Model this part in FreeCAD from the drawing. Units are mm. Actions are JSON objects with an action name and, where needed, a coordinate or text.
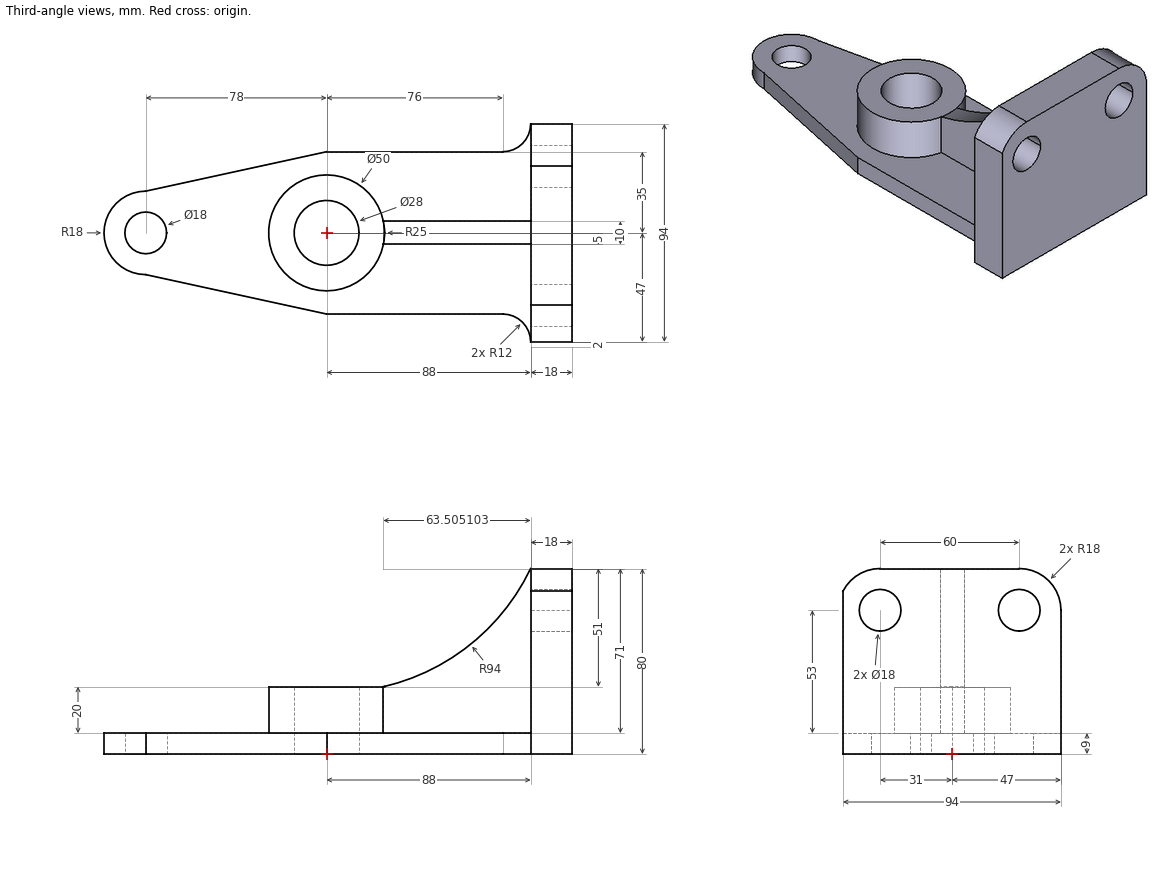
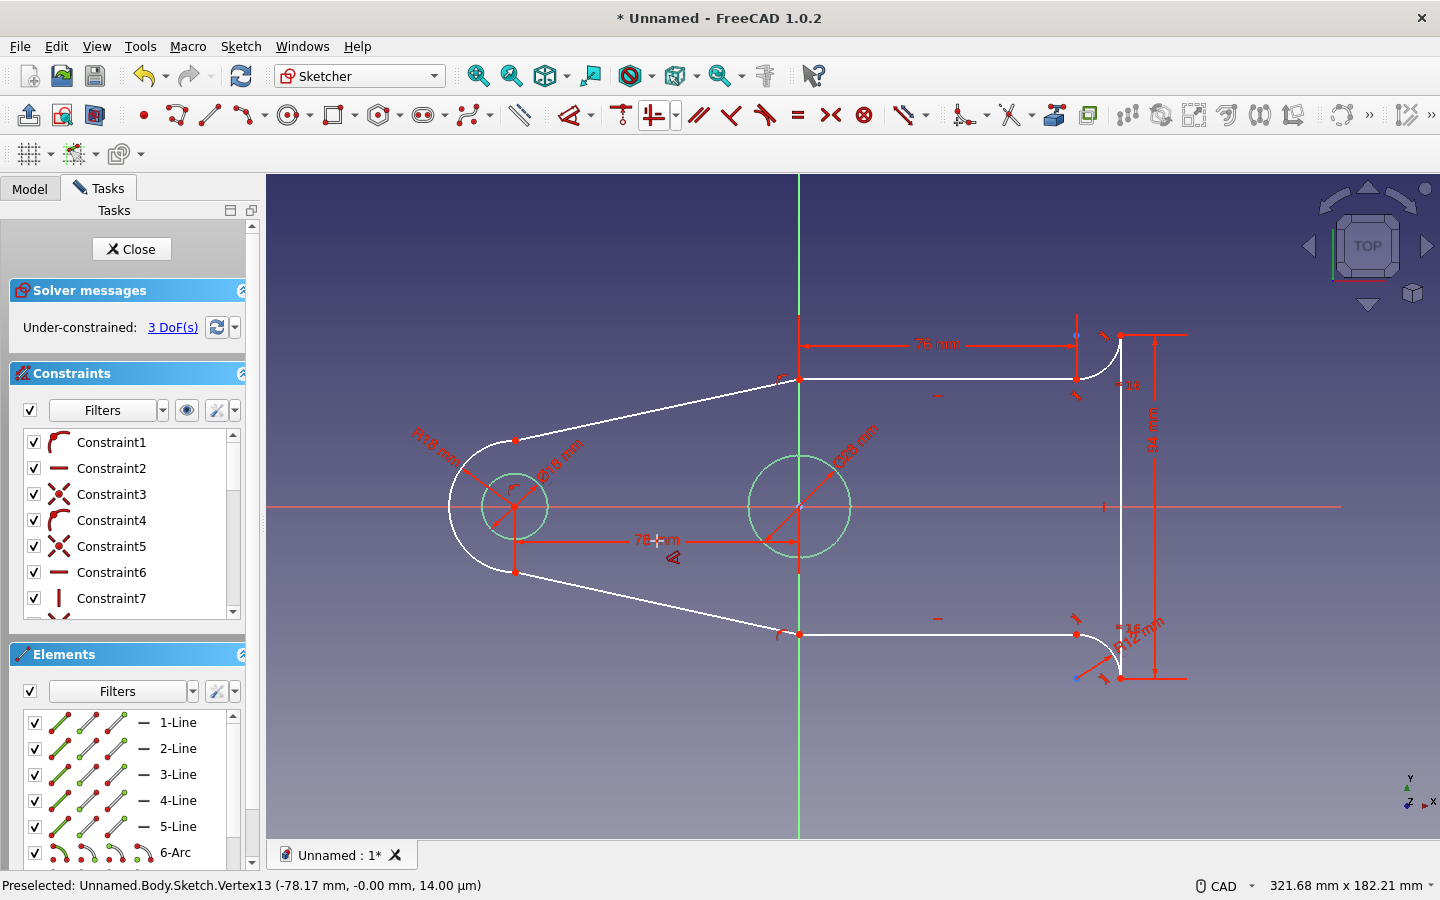
{"action": "left_click", "coordinate": [1077, 379]}
{"action": "left_click", "coordinate": [765, 443]}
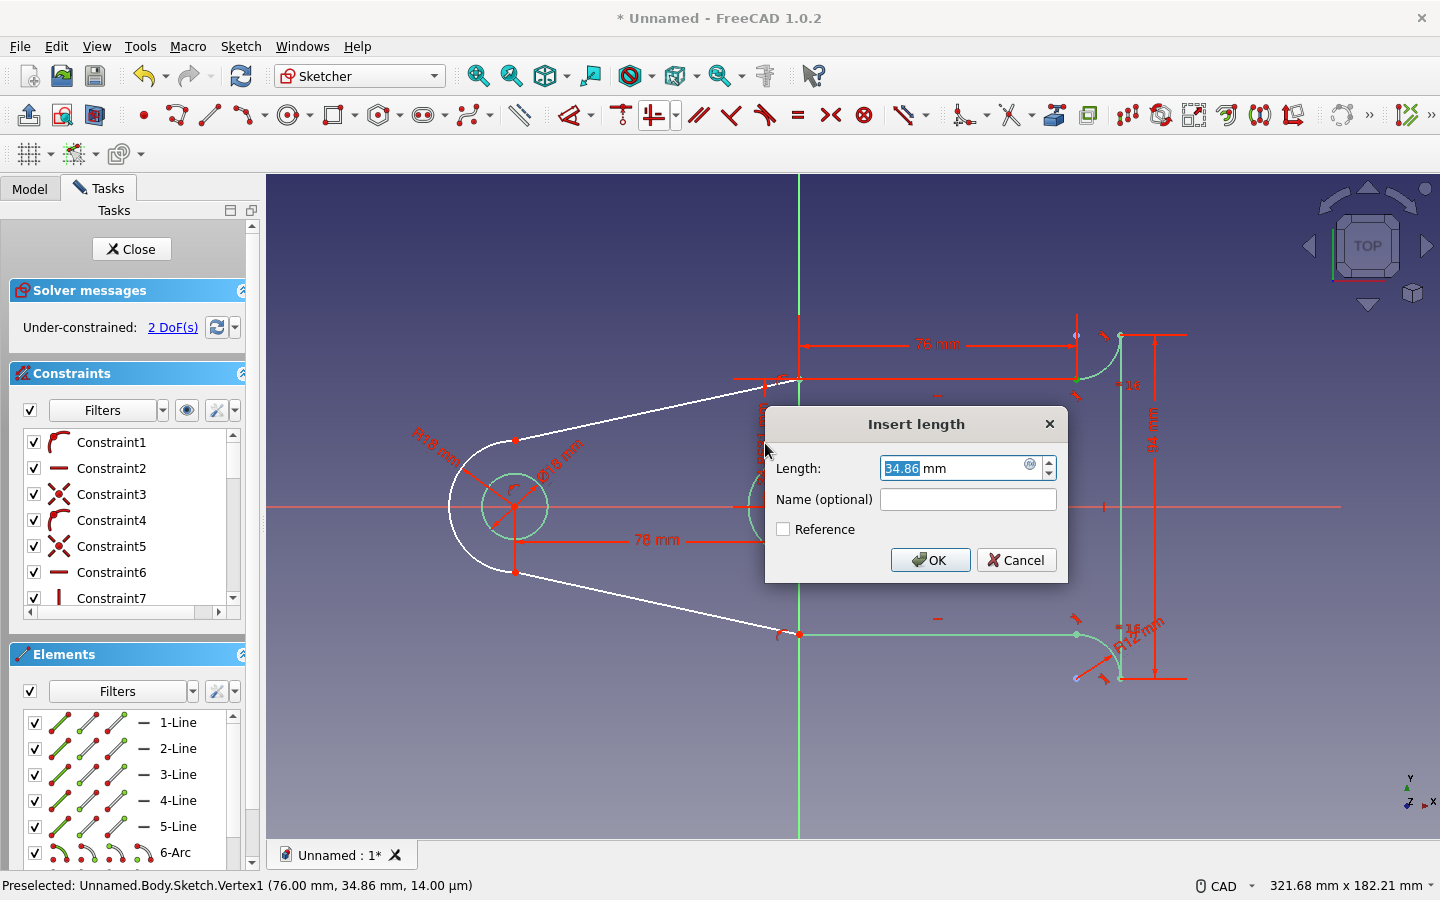
{"action": "type", "text": "35"}
{"action": "key", "text": "Return"}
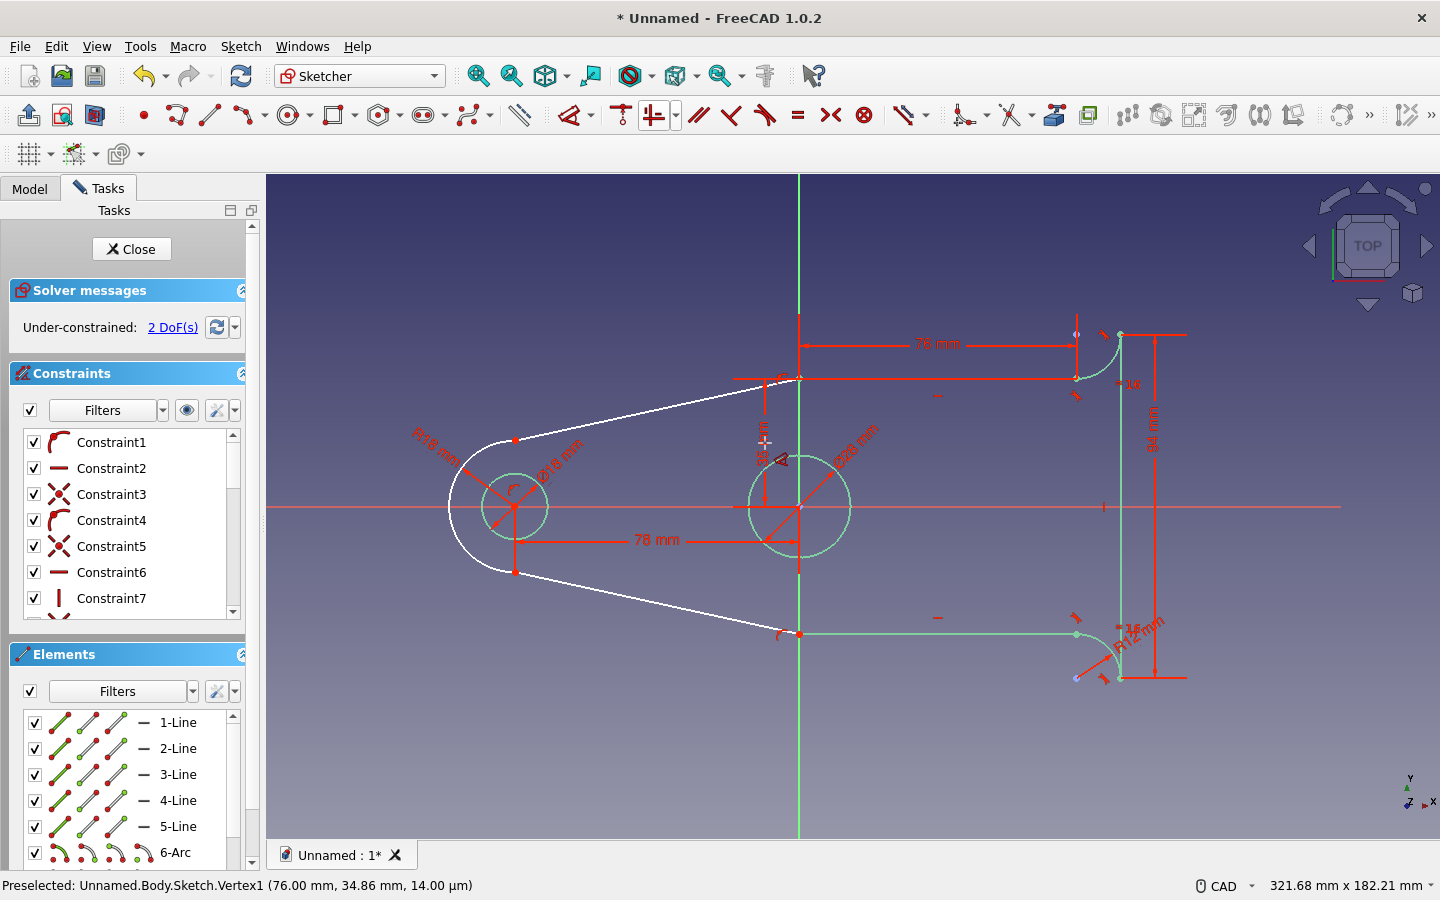
{"action": "left_click", "coordinate": [515, 441]}
{"action": "left_click", "coordinate": [592, 407]}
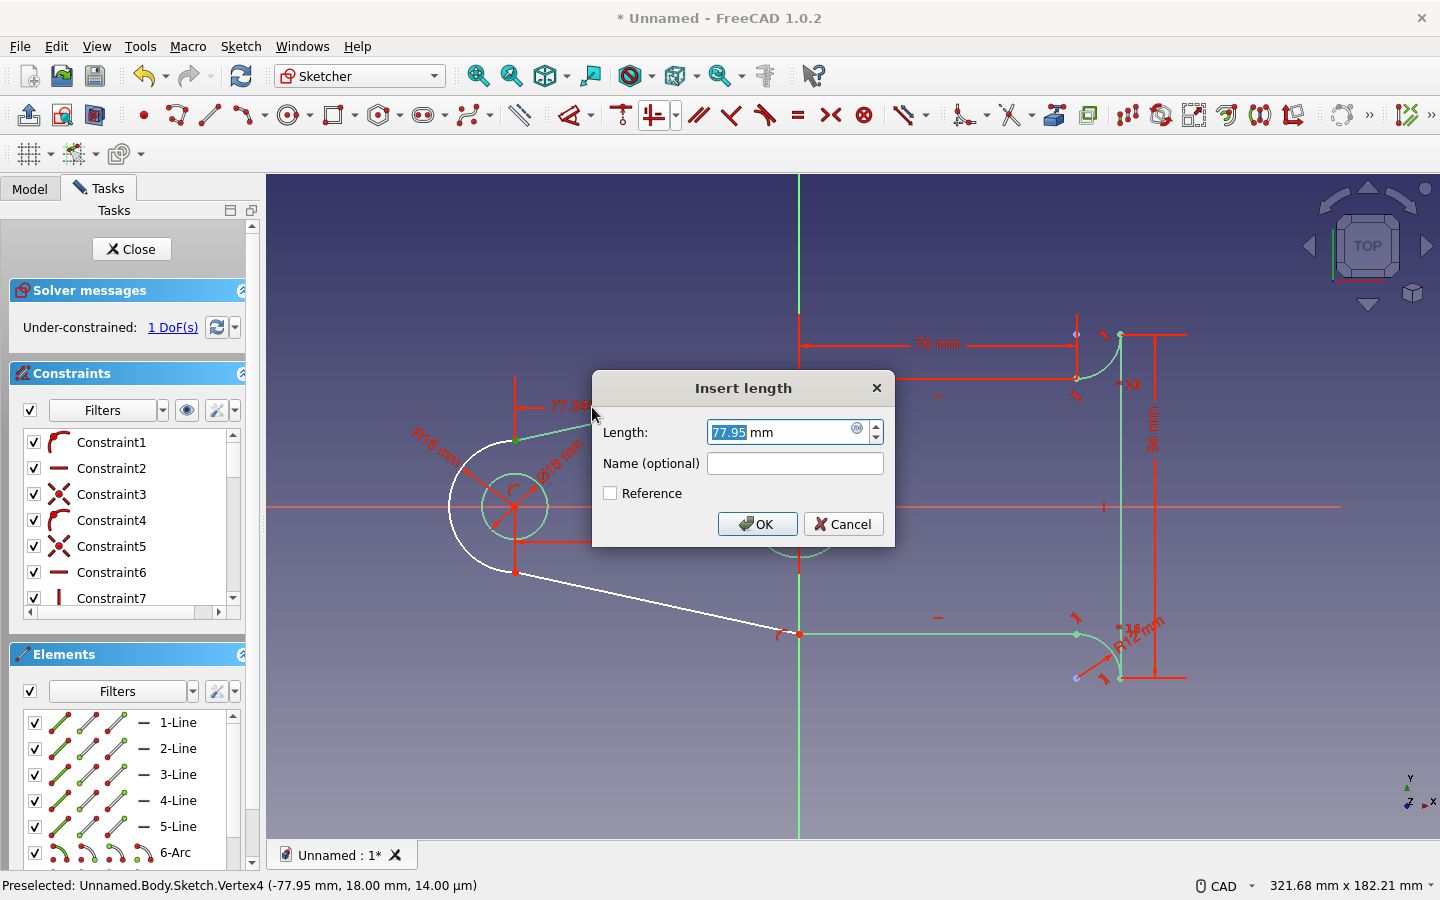
{"action": "type", "text": "78"}
{"action": "key", "text": "Return"}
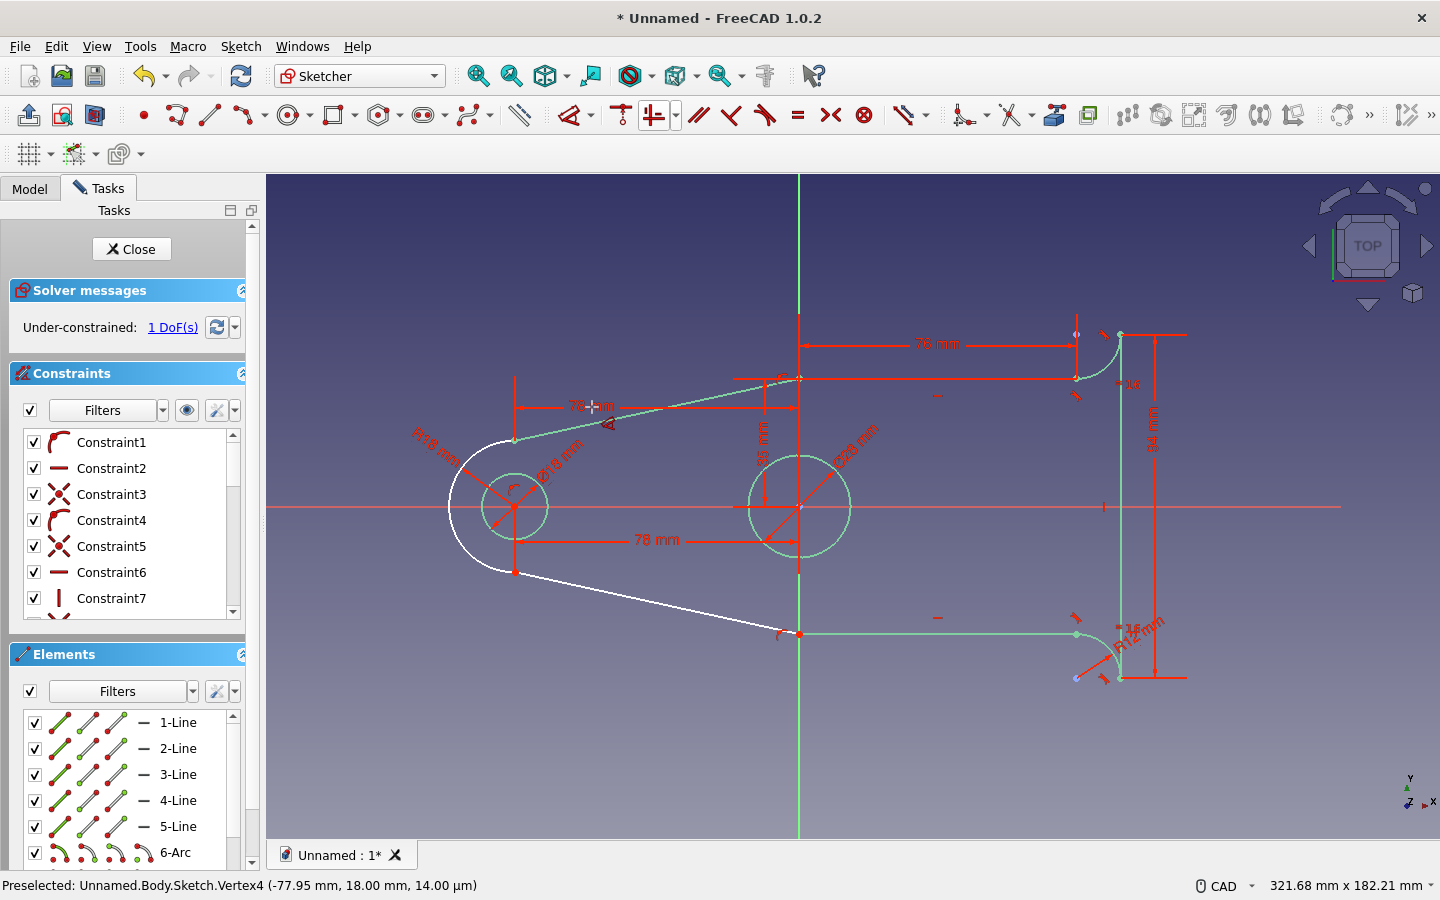
{"action": "left_click", "coordinate": [515, 572]}
{"action": "left_click", "coordinate": [592, 606]}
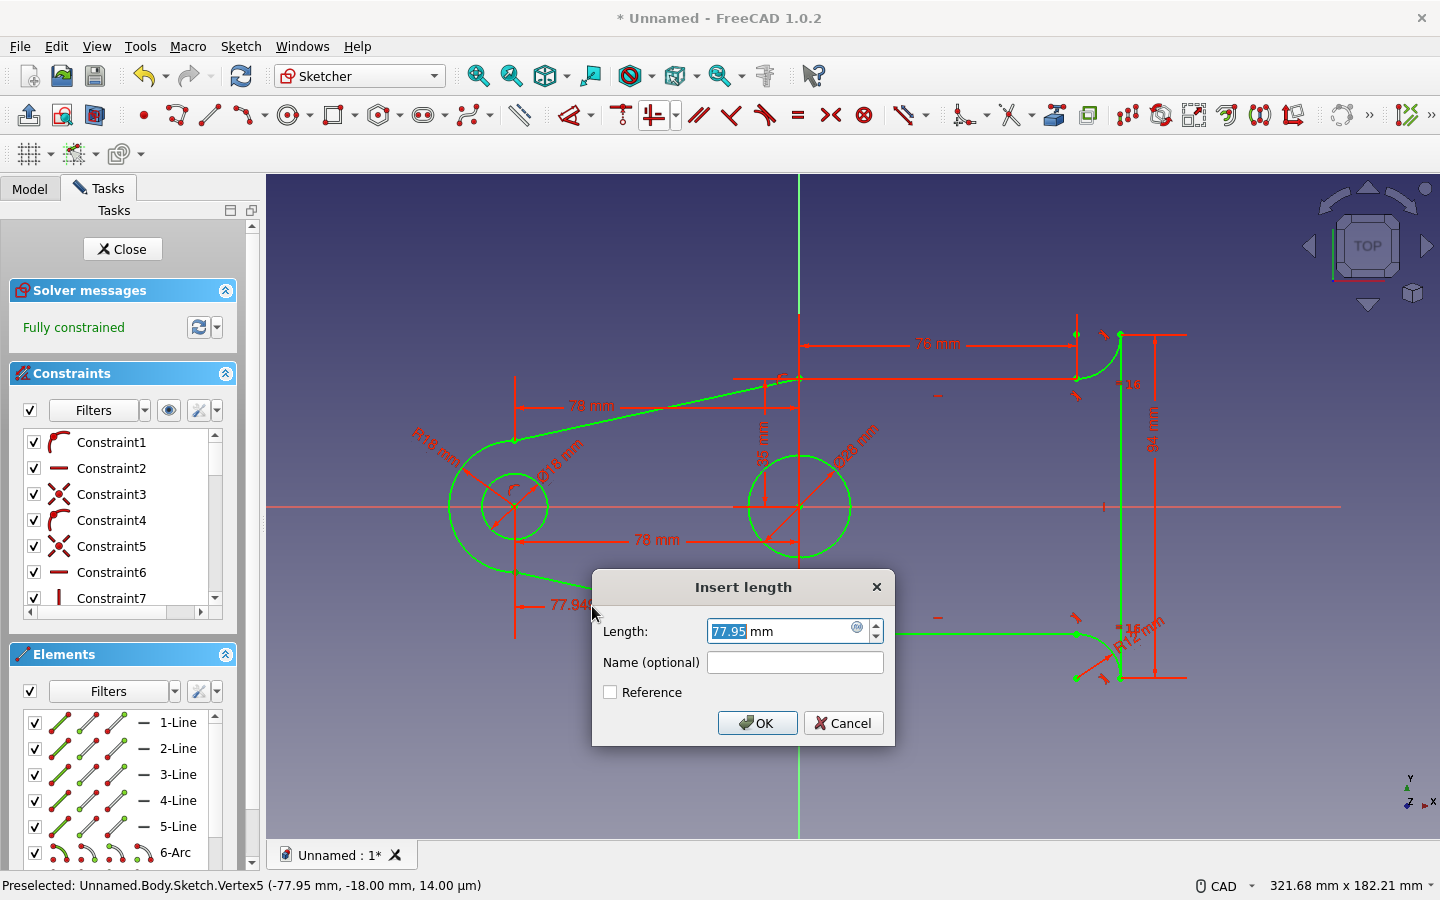
{"action": "type", "text": "78"}
{"action": "key", "text": "Return"}
{"action": "key", "text": "Escape"}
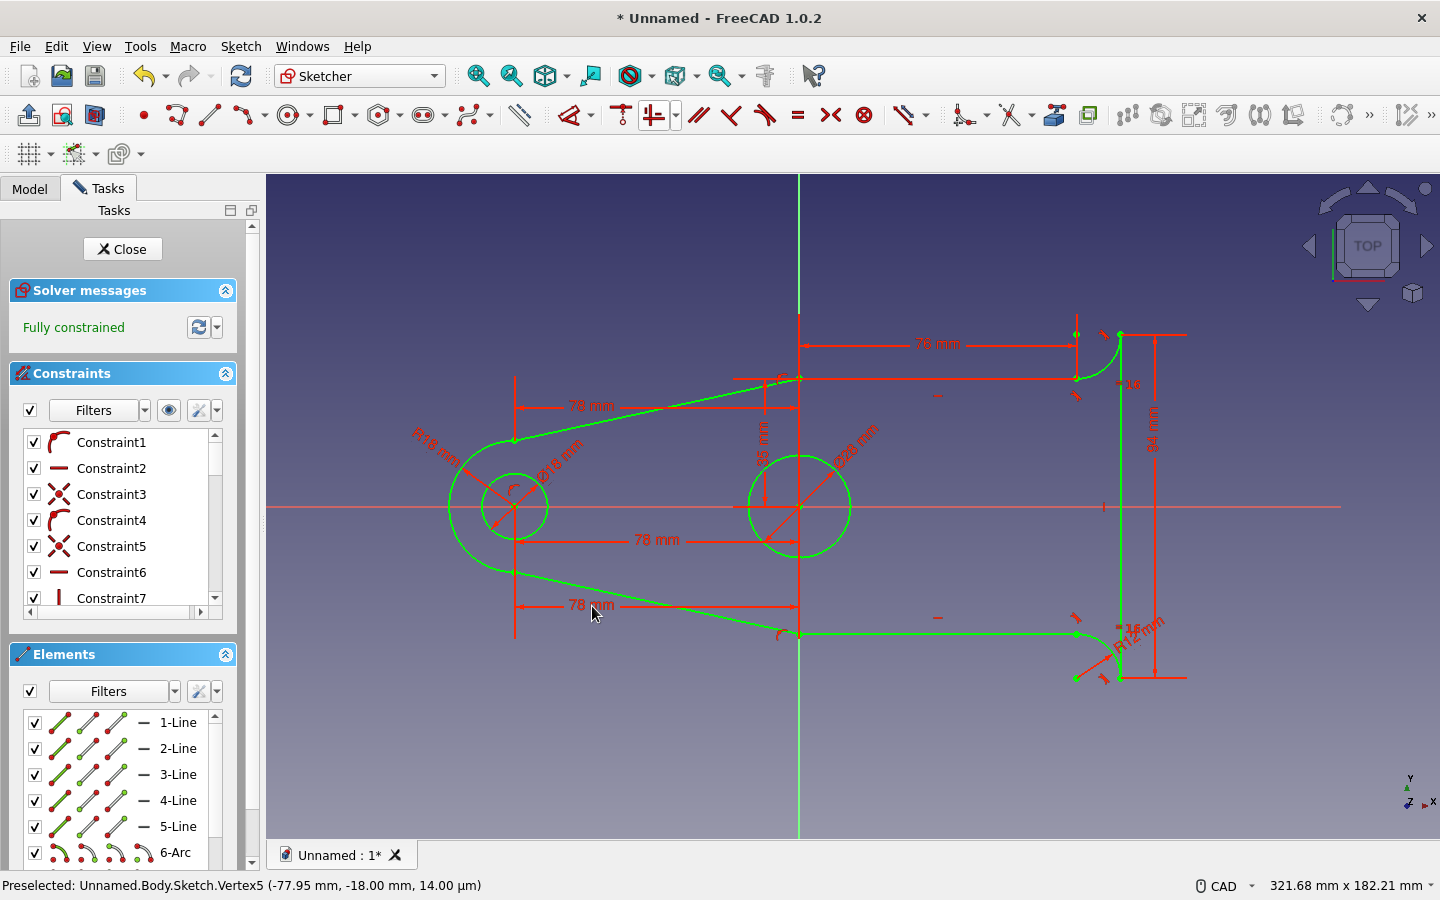
{"action": "left_click", "coordinate": [123, 249]}